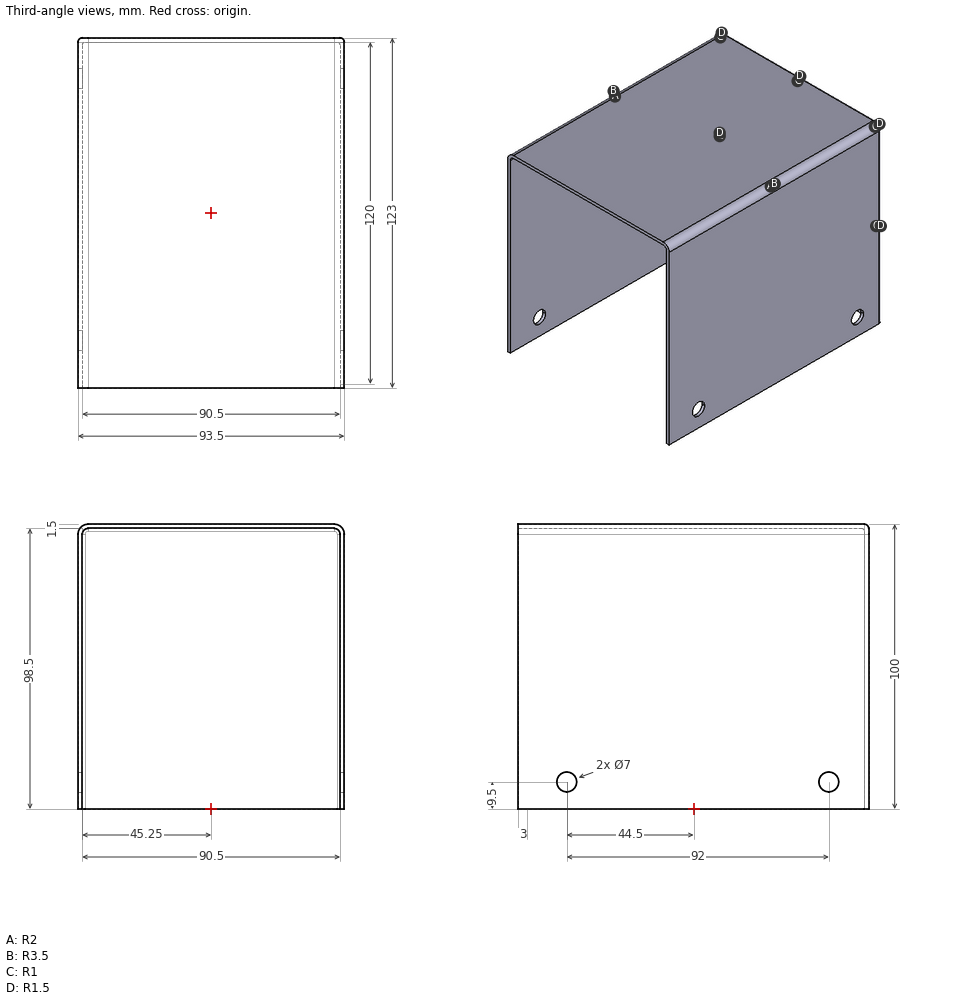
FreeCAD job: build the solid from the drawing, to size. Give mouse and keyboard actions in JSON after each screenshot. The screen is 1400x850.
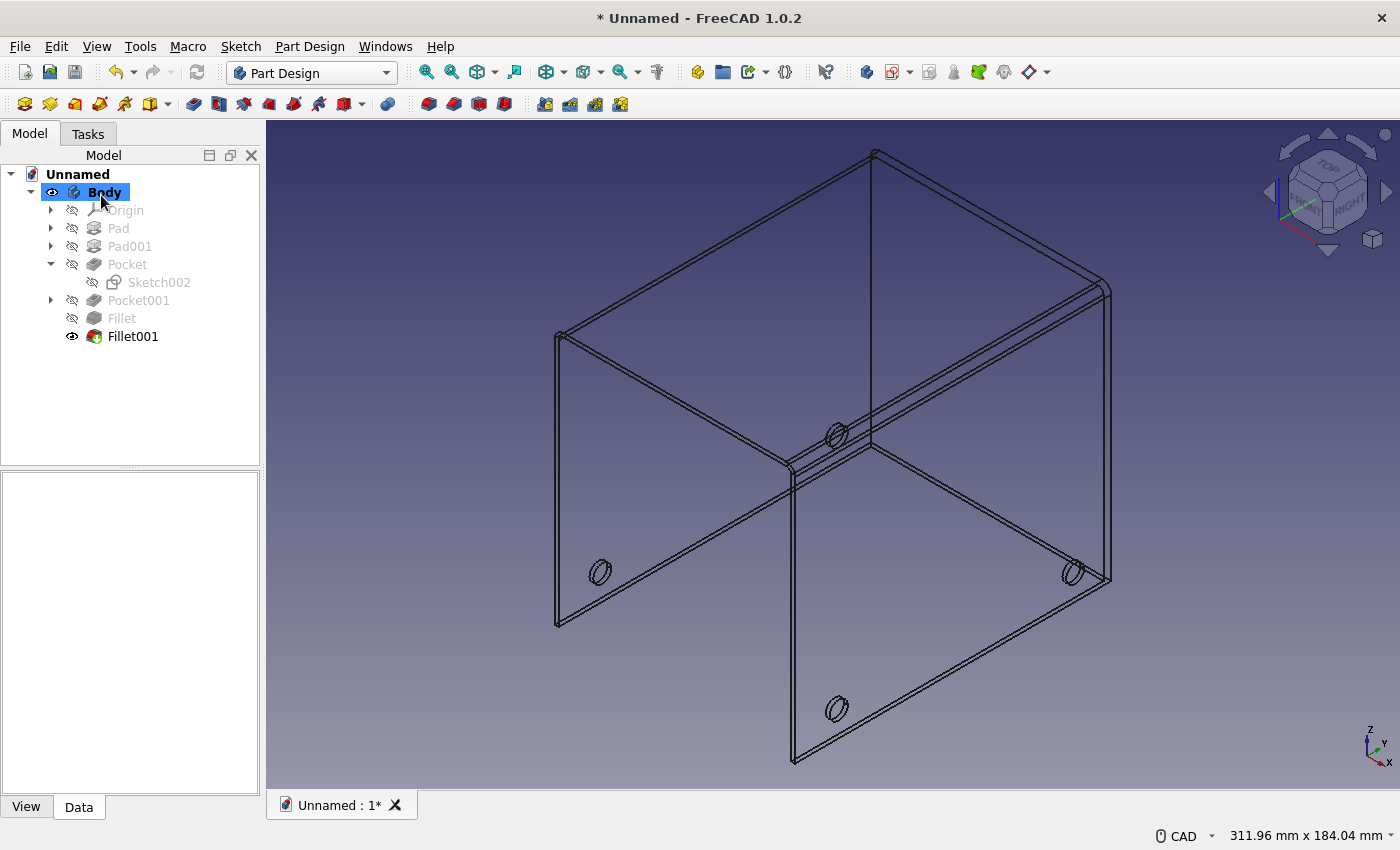
{"action": "left_click", "coordinate": [871, 303]}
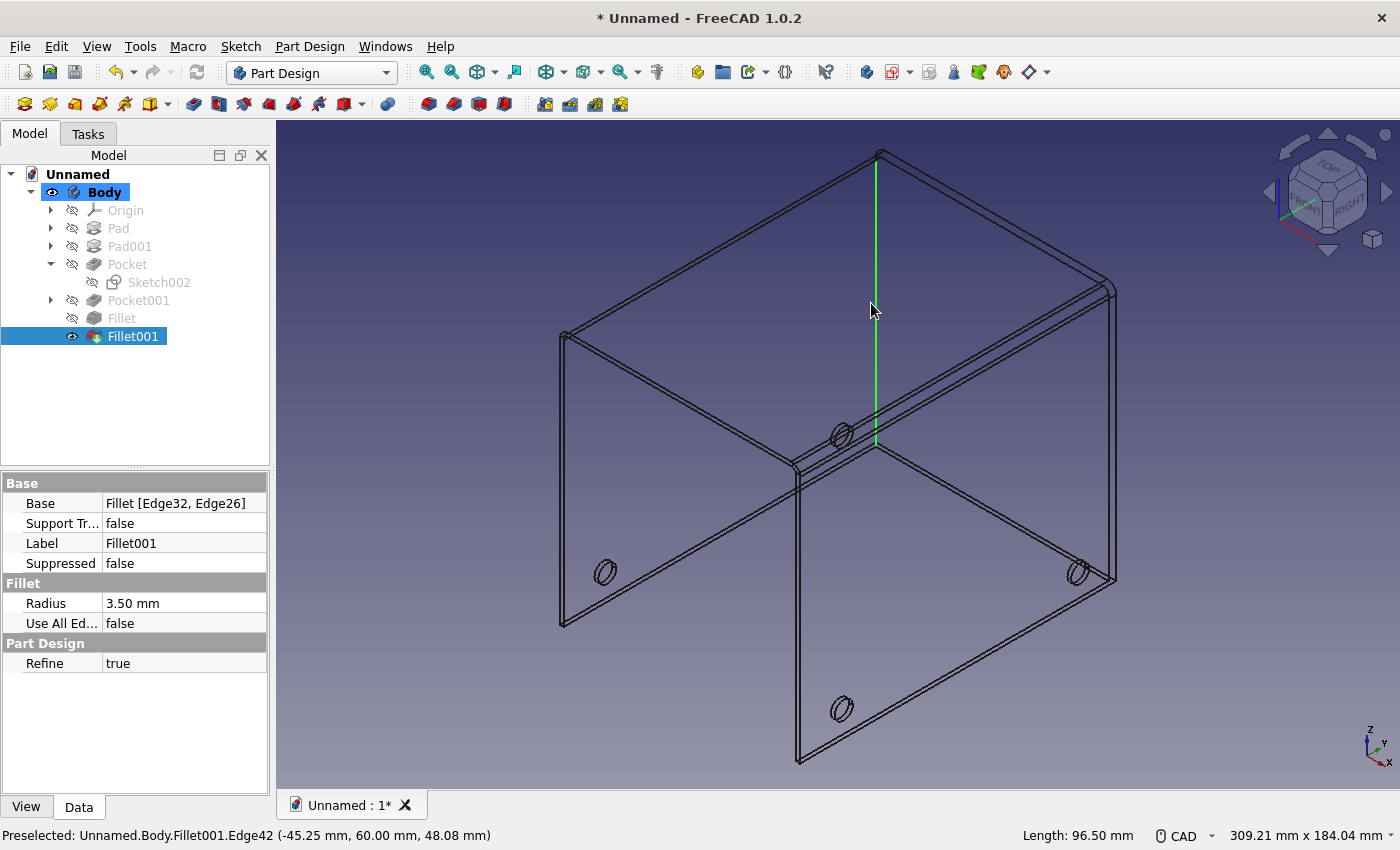
{"action": "left_click", "coordinate": [992, 221], "text": "ctrl"}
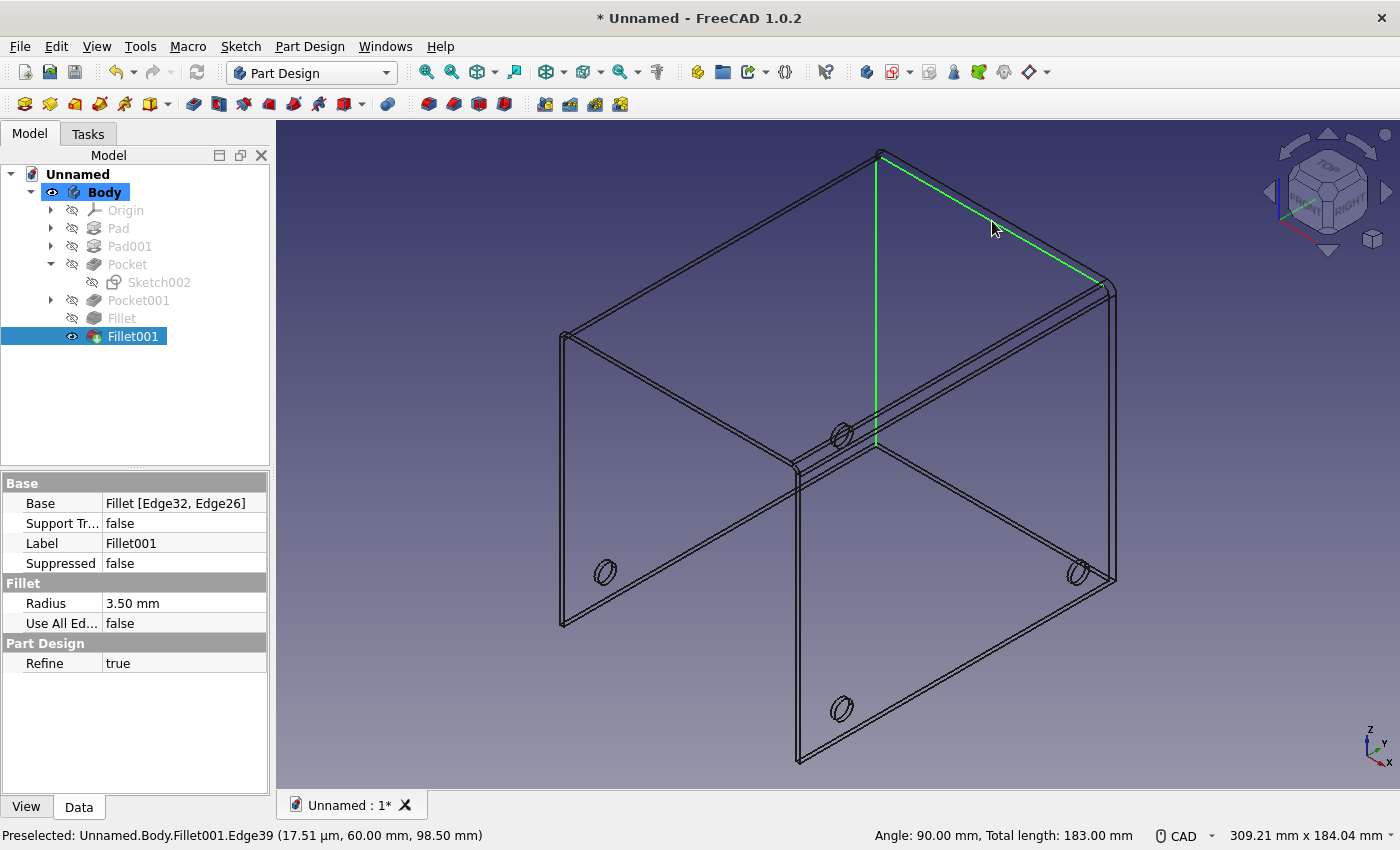
{"action": "left_click", "coordinate": [1109, 437], "text": "ctrl"}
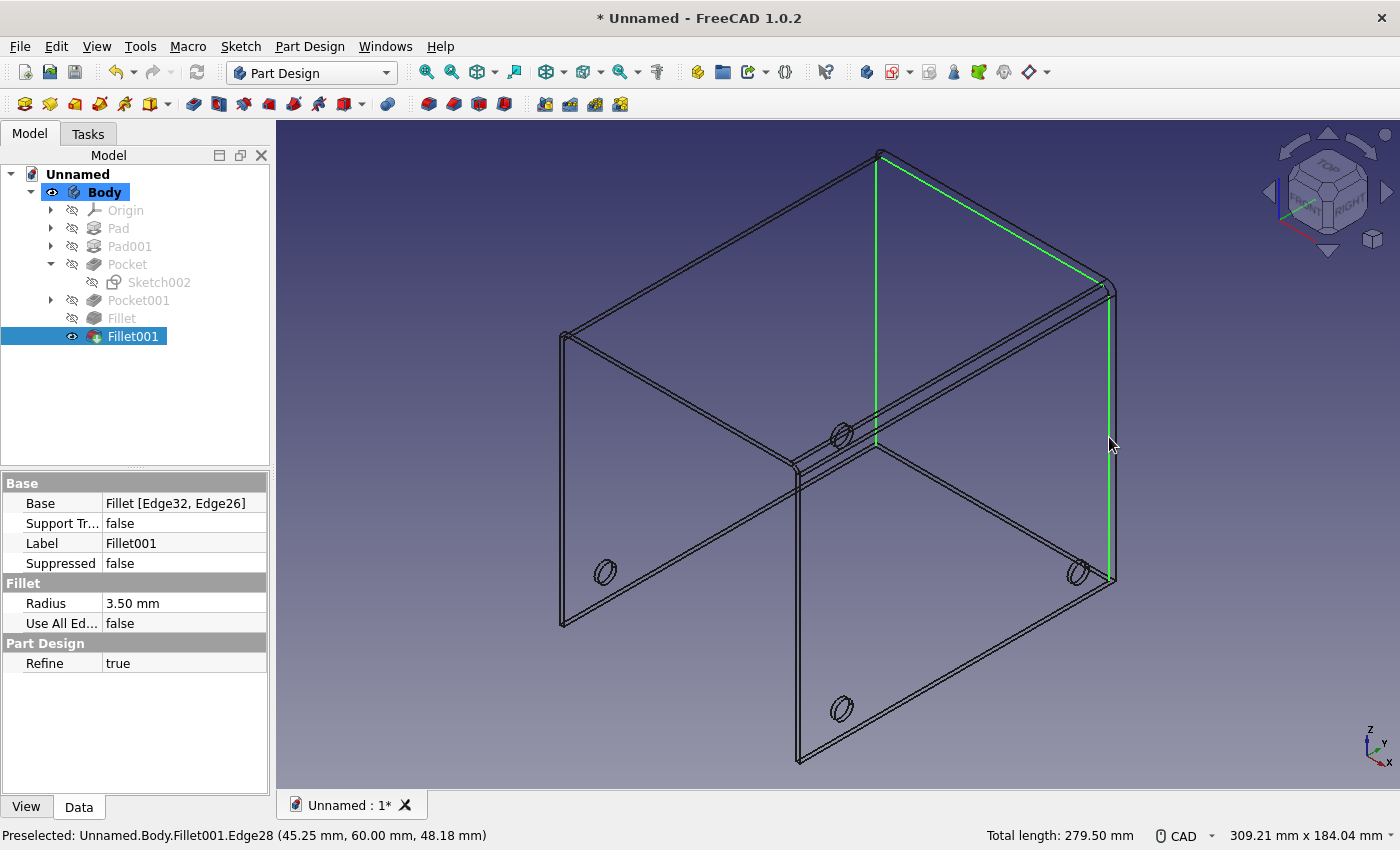
{"action": "left_click", "coordinate": [1107, 289], "text": "ctrl"}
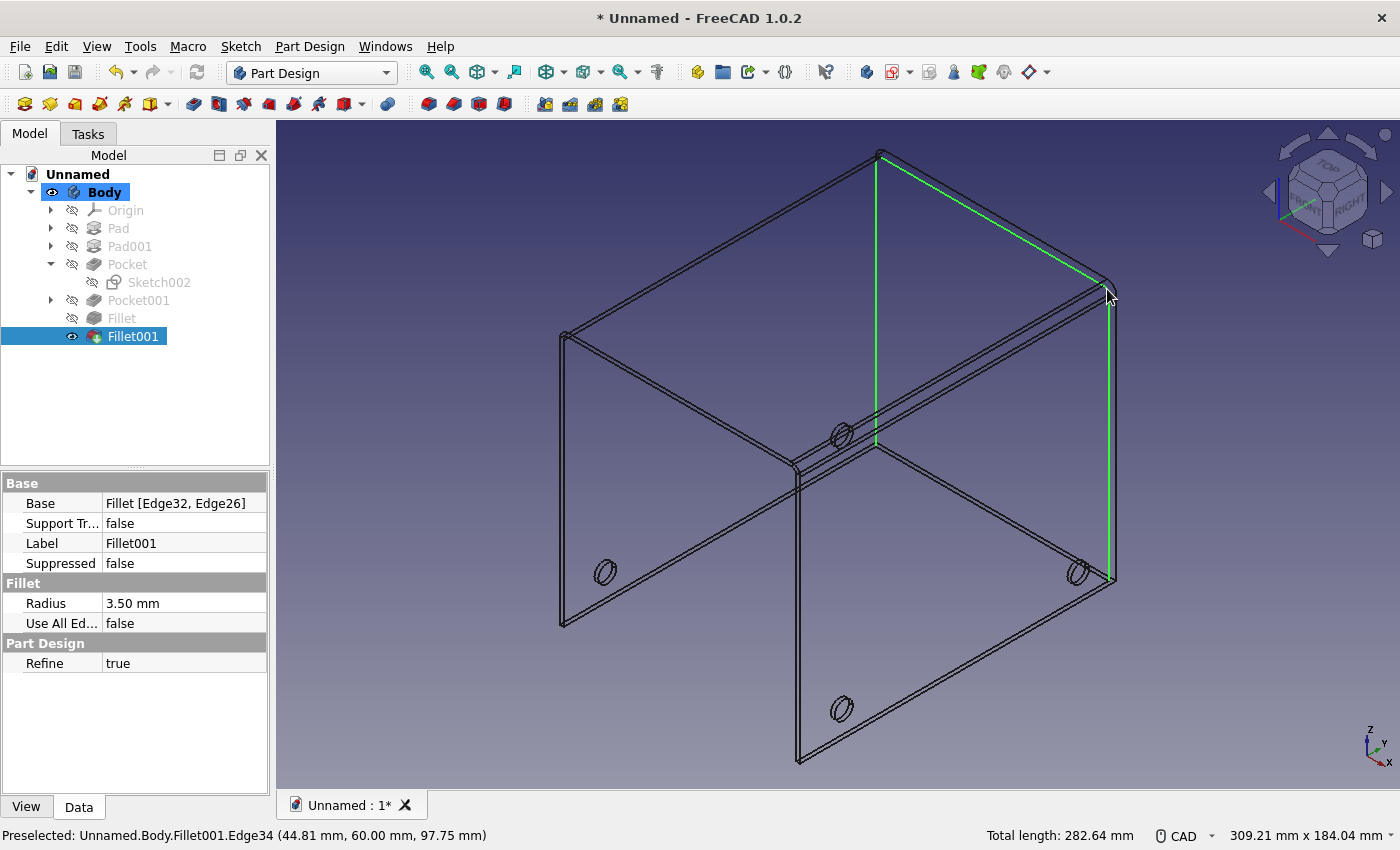
{"action": "scroll", "coordinate": [877, 156], "scroll_direction": "up", "scroll_amount": 7}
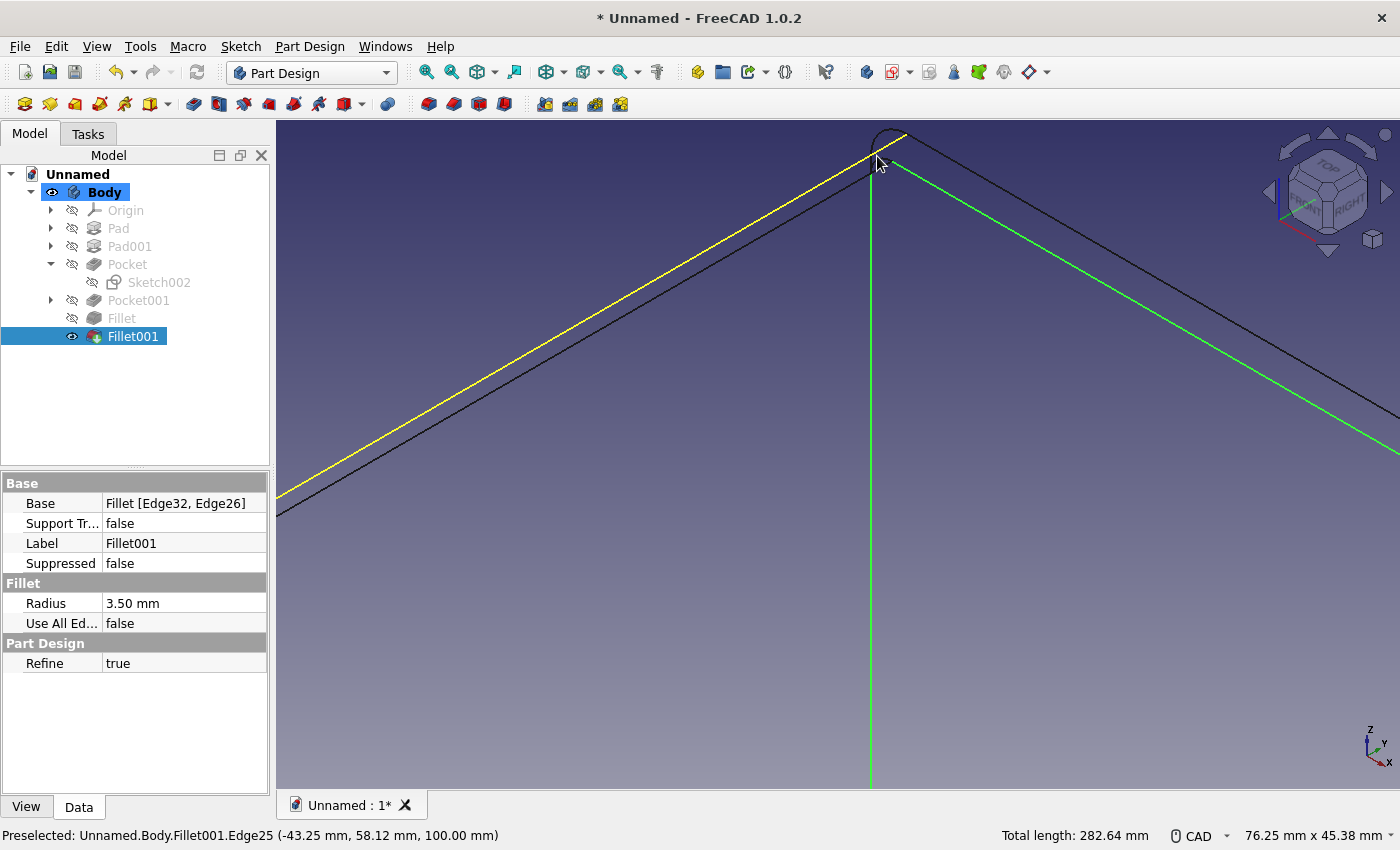
{"action": "left_click", "coordinate": [877, 159], "text": "ctrl"}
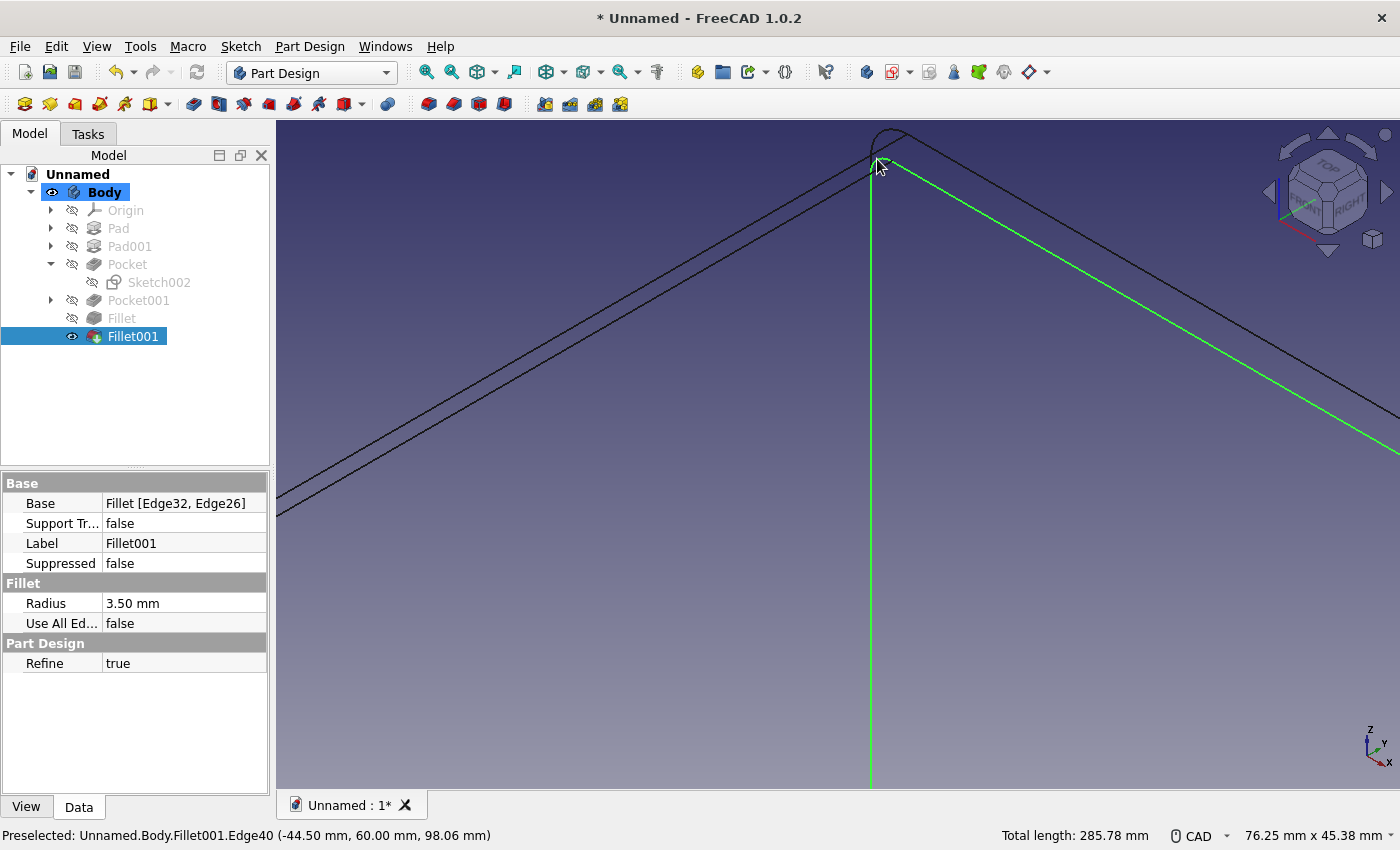
{"action": "key", "text": "v 1"}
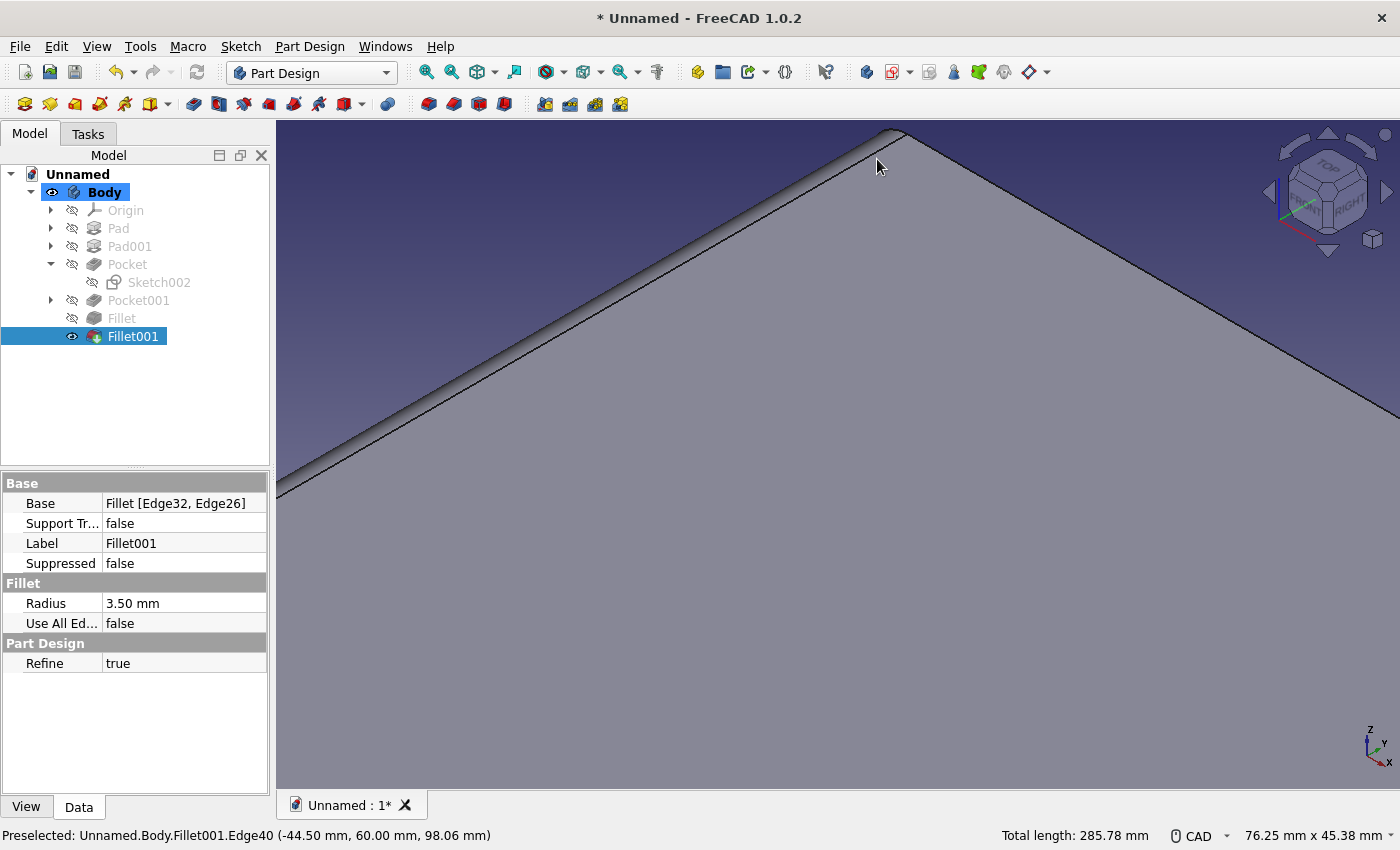
{"action": "left_click", "coordinate": [429, 104]}